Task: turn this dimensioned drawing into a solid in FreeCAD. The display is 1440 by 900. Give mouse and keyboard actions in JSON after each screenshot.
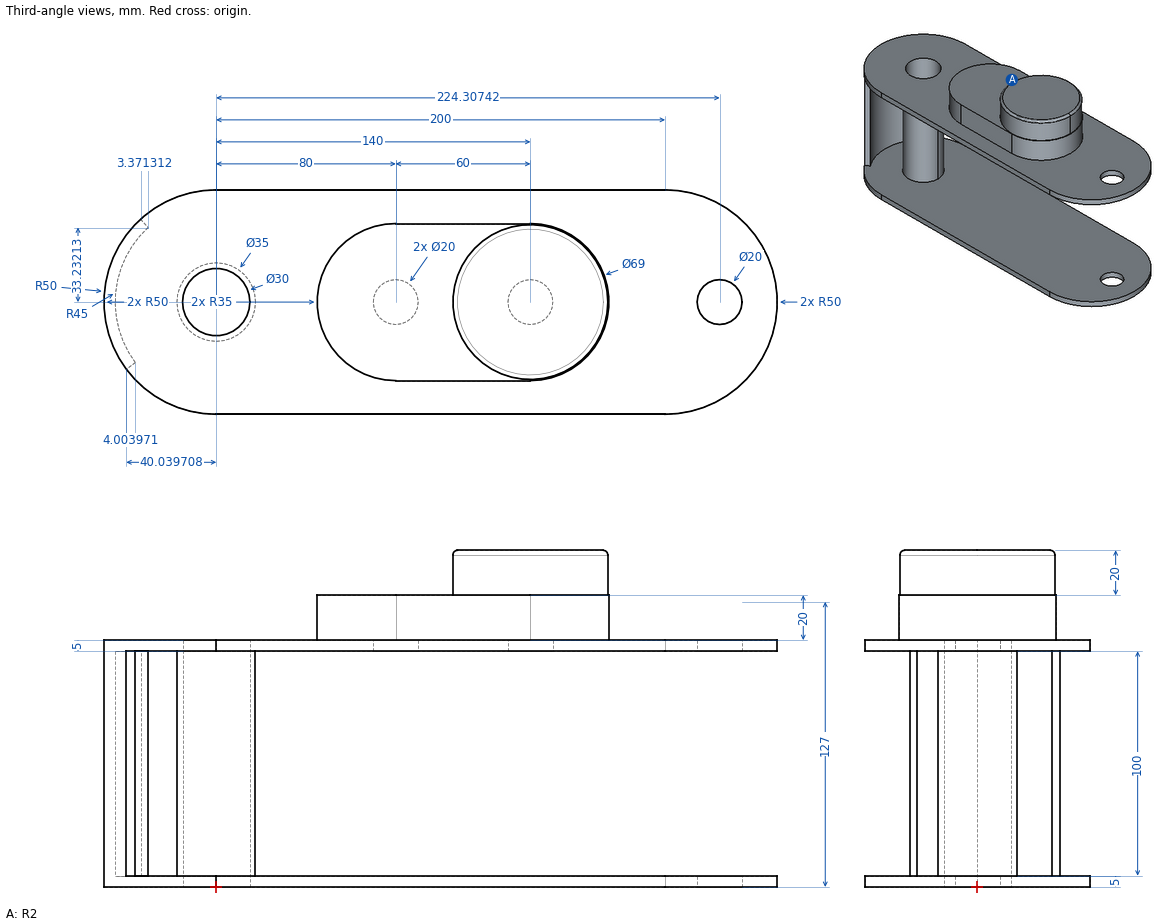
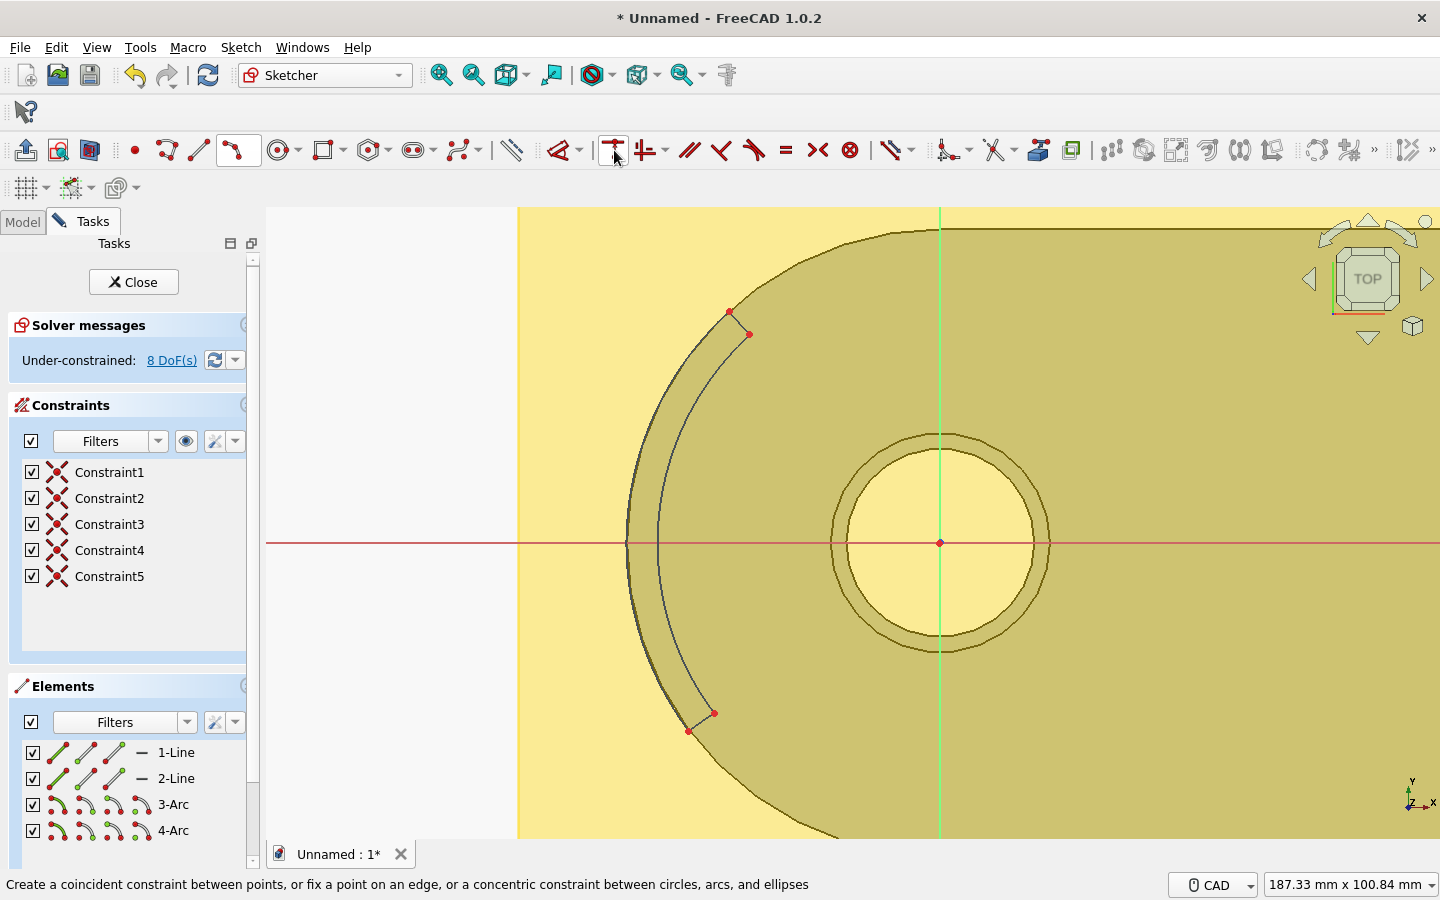
{"action": "left_click_drag", "start_coordinate": [930, 533], "coordinate": [950, 554]}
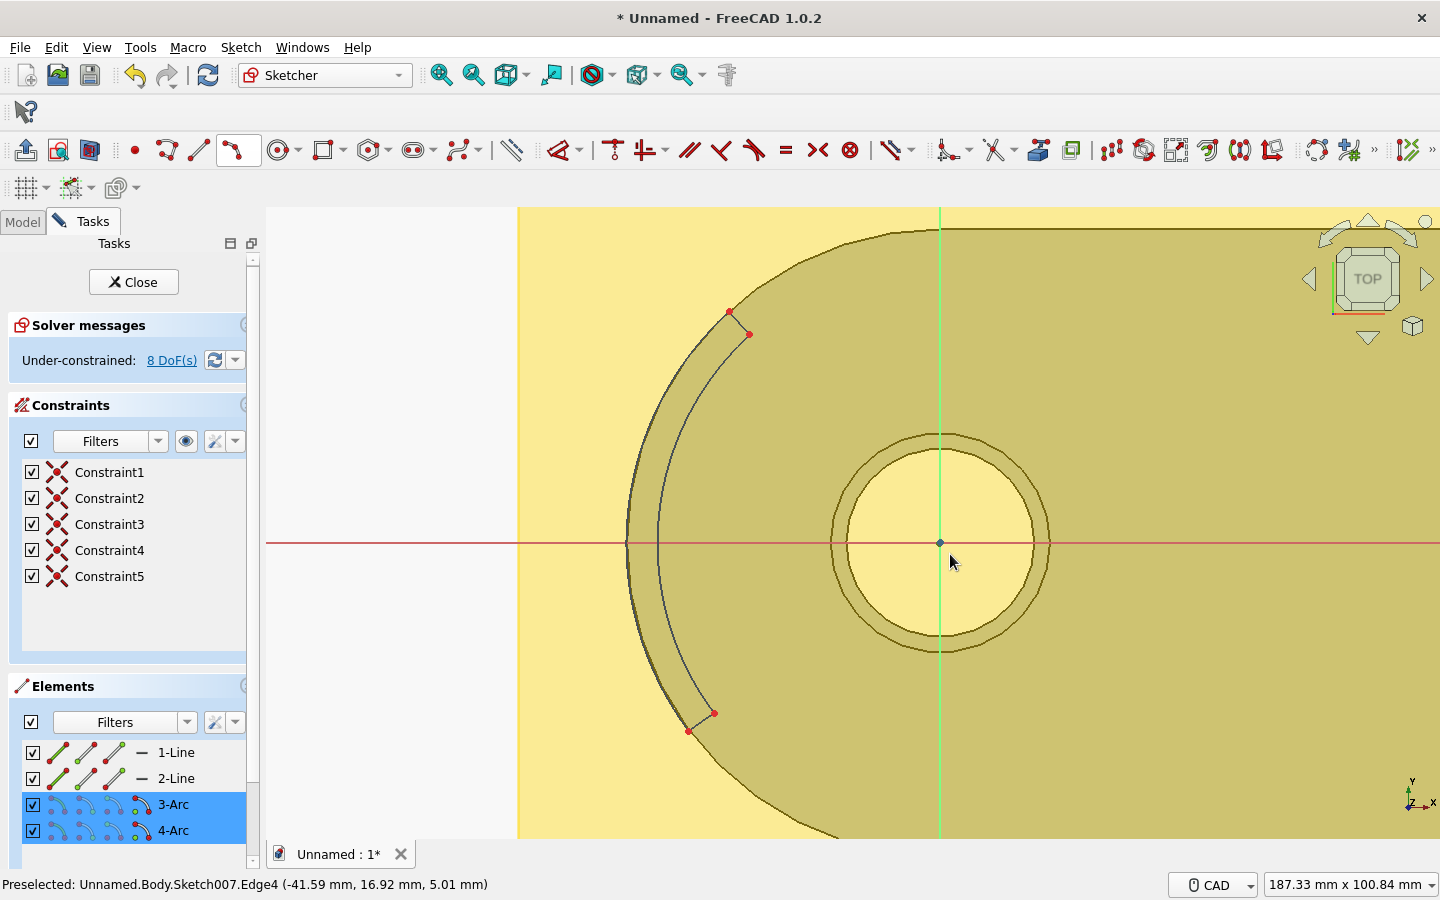
{"action": "left_click", "coordinate": [614, 150]}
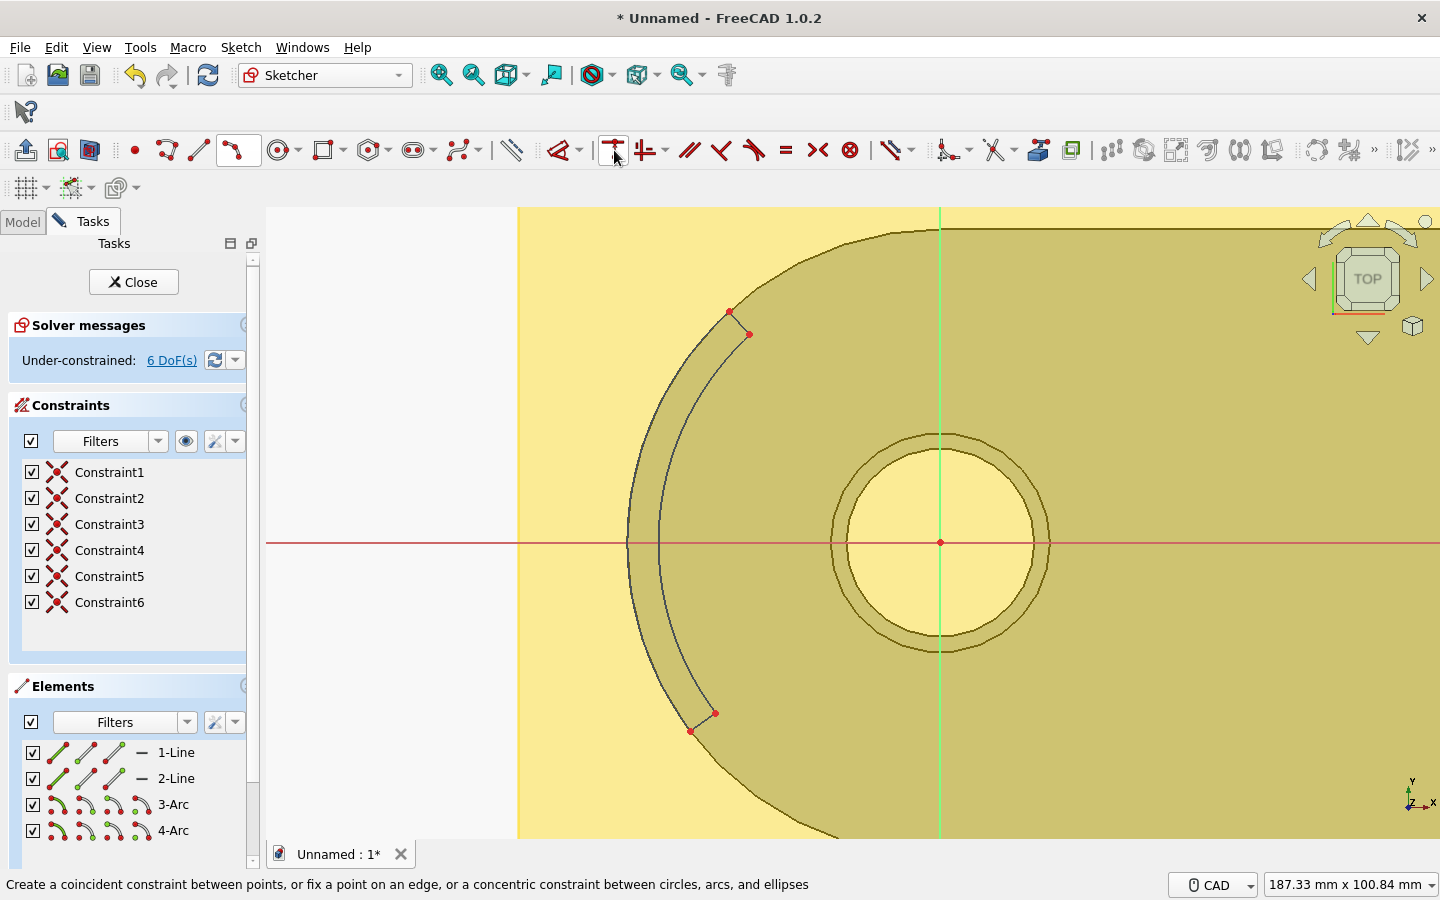
{"action": "left_click", "coordinate": [558, 150]}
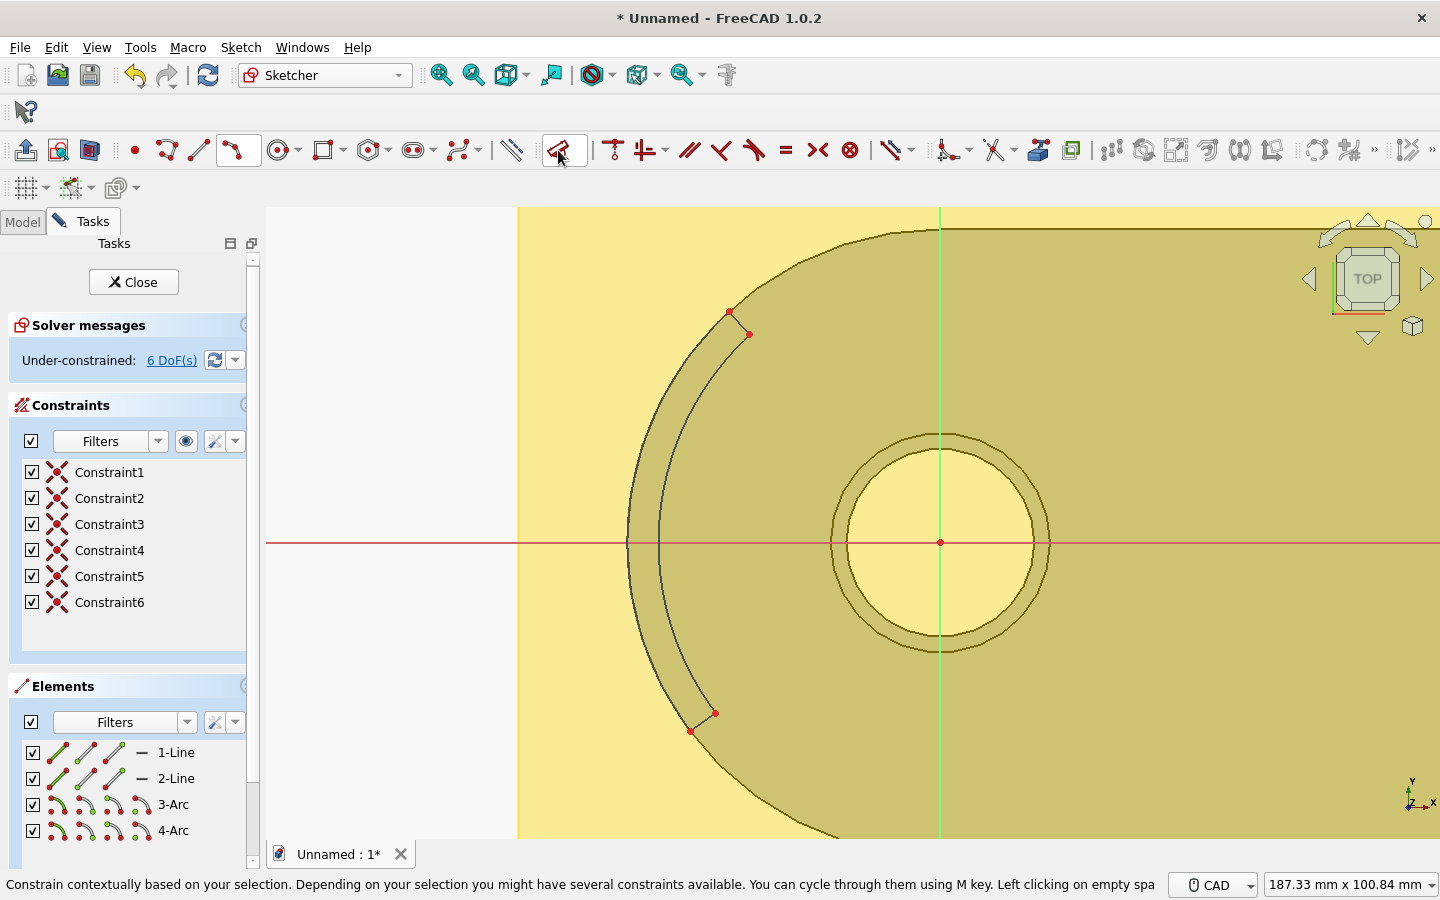
{"action": "left_click", "coordinate": [651, 425]}
{"action": "left_click", "coordinate": [621, 413]}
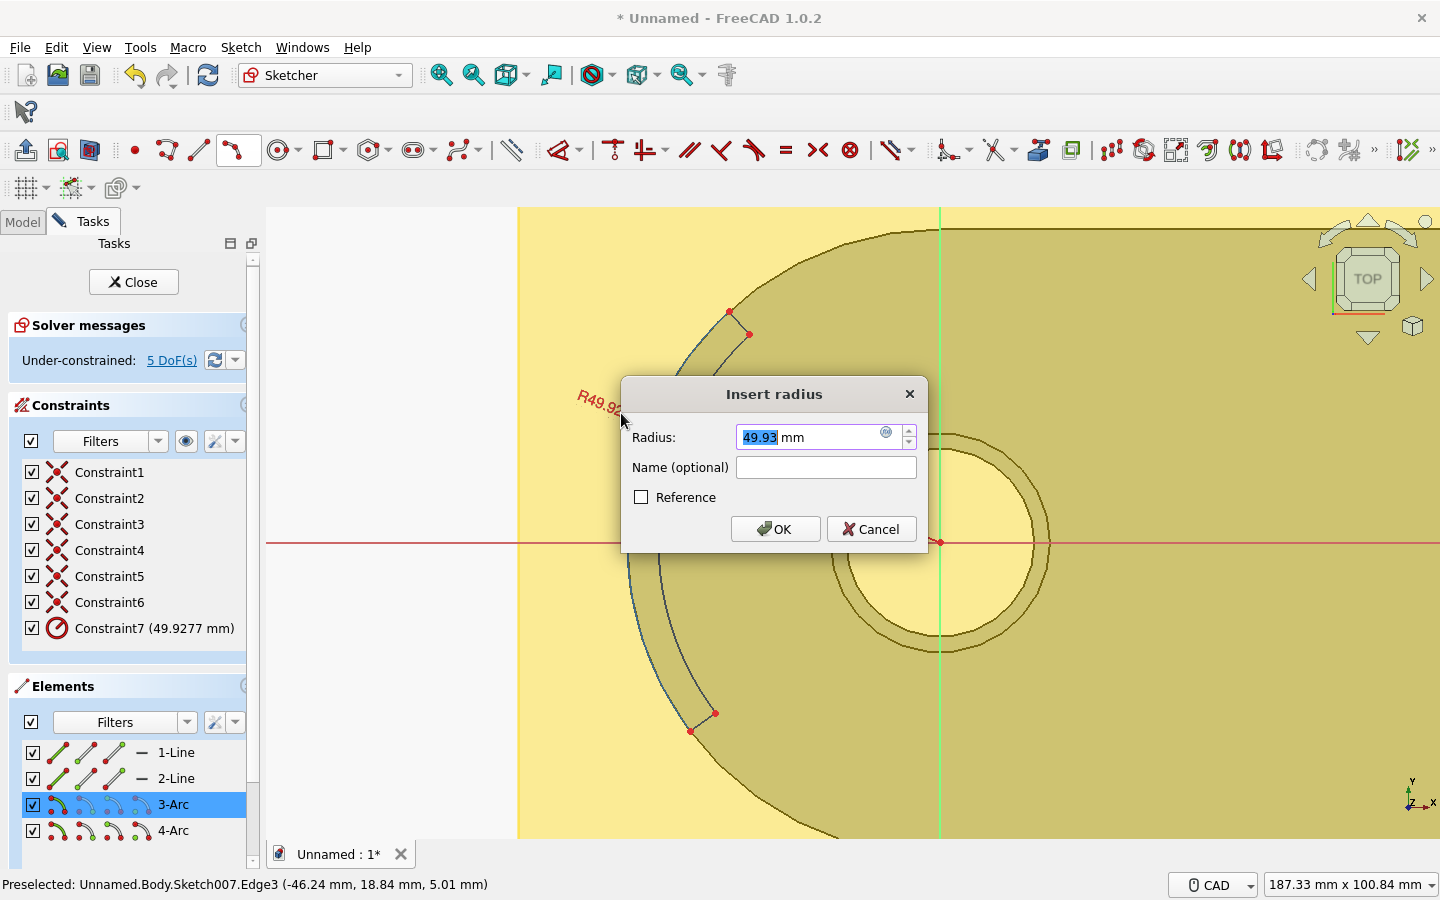
{"action": "type", "text": "50"}
{"action": "key", "text": "Return"}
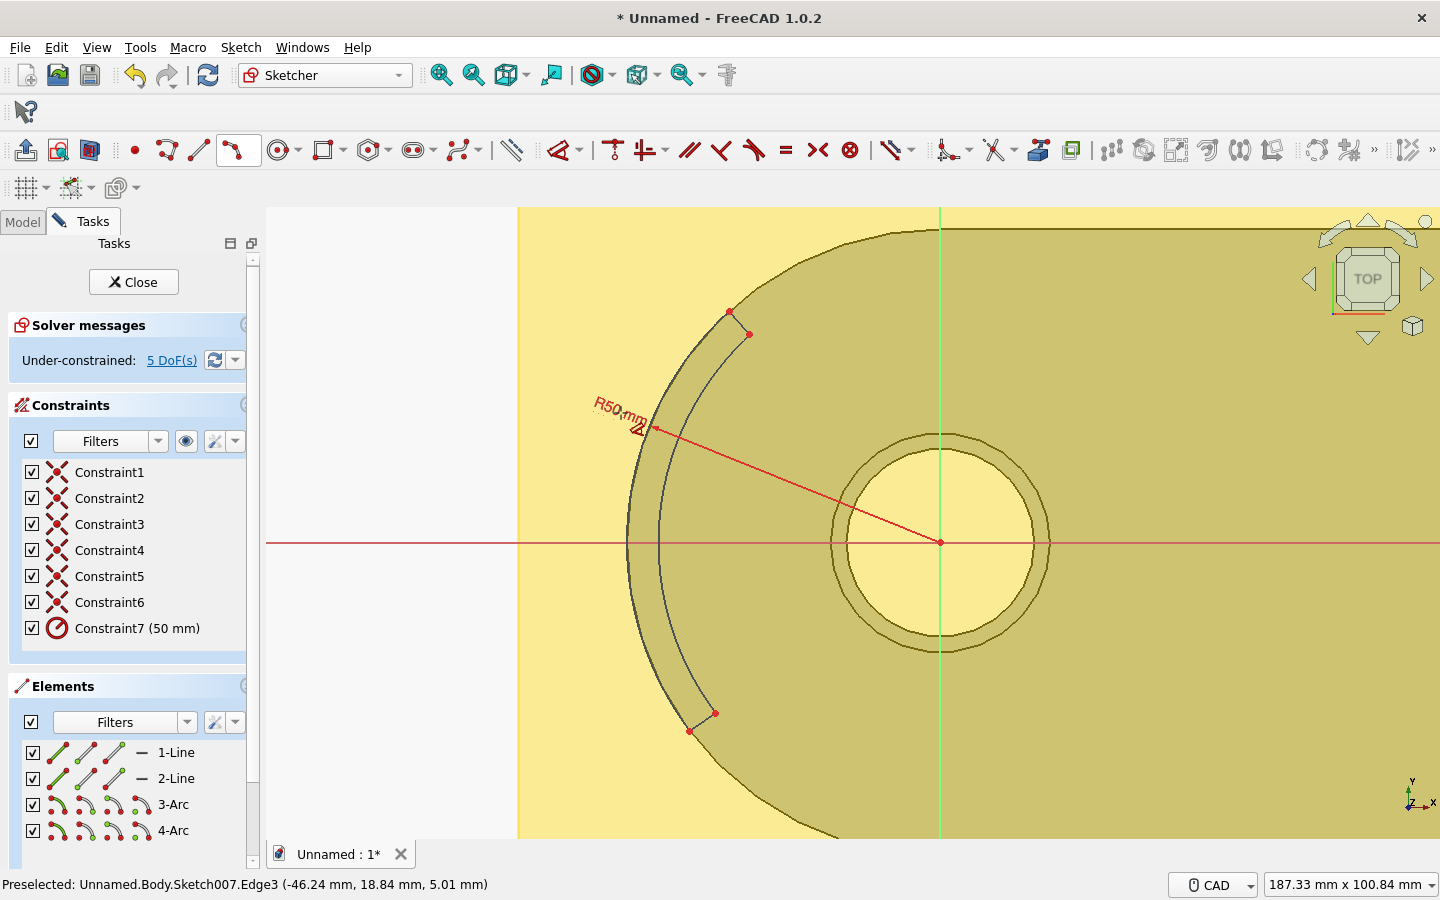
{"action": "left_click", "coordinate": [679, 437]}
{"action": "left_click", "coordinate": [741, 300]}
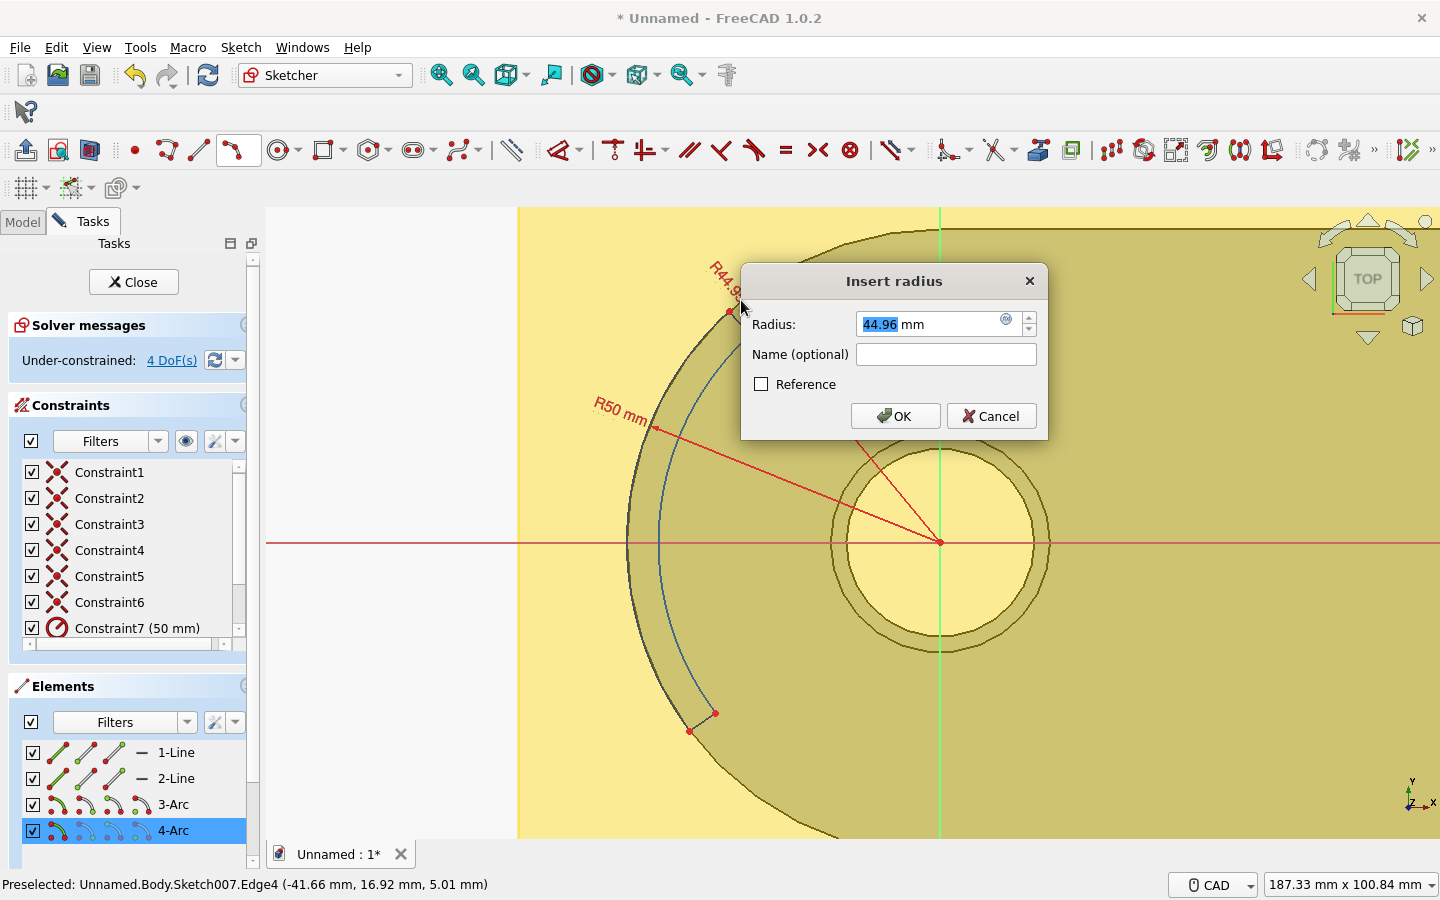
{"action": "type", "text": "45"}
{"action": "key", "text": "Return"}